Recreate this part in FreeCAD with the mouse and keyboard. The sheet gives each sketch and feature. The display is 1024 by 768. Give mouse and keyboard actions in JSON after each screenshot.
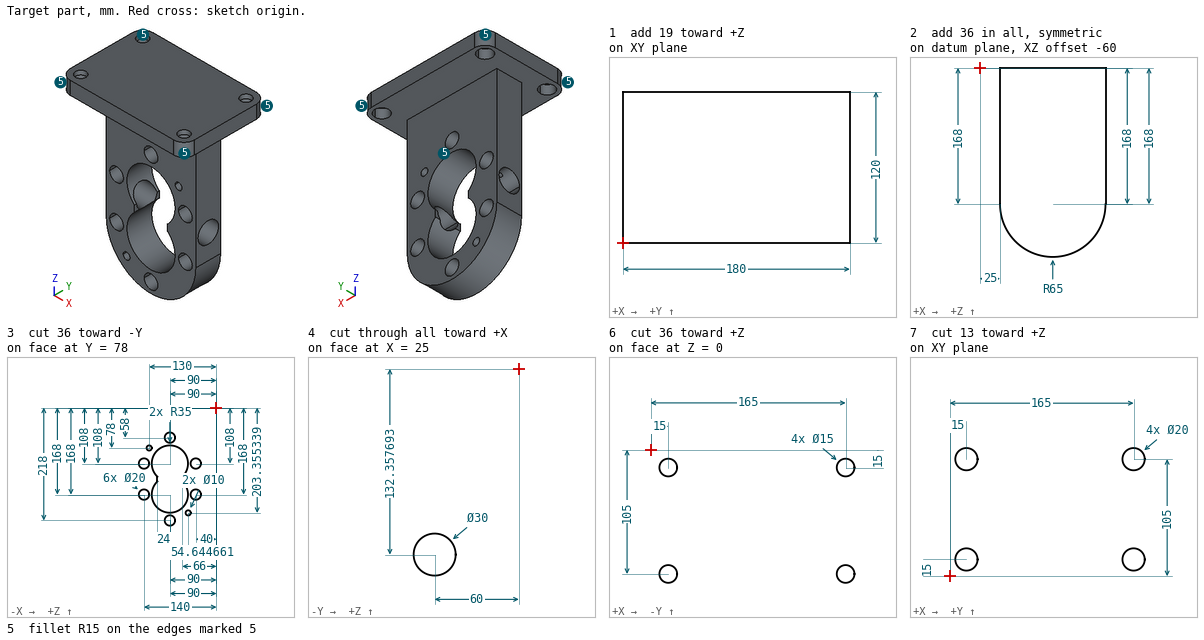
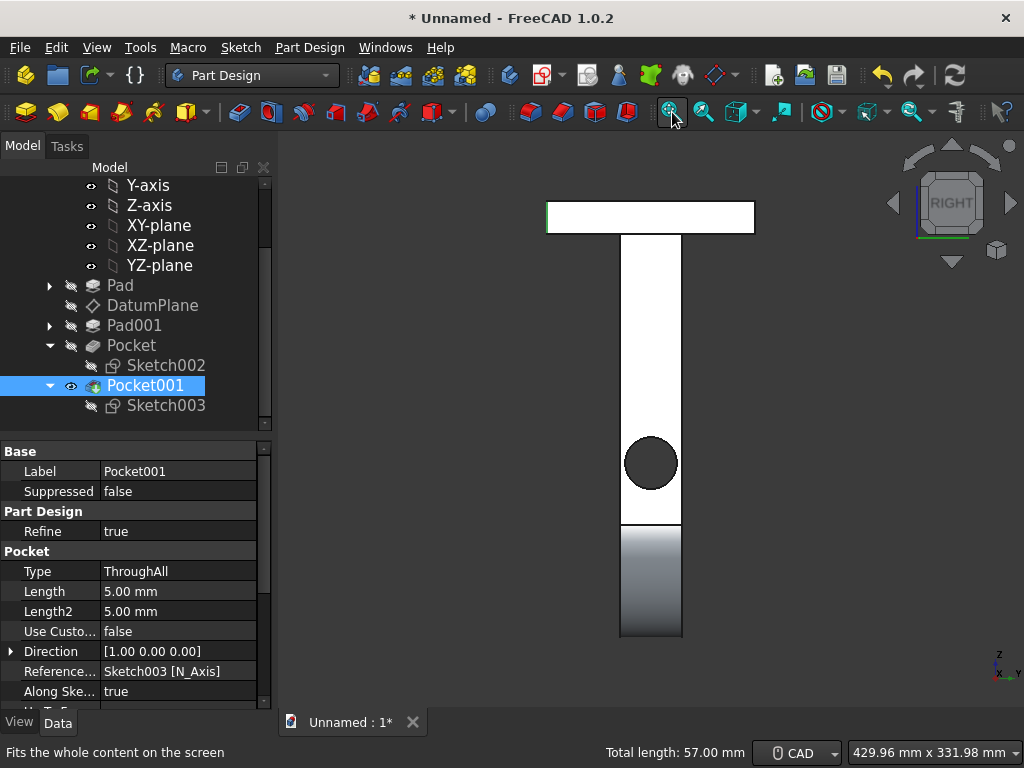
{"action": "left_click", "coordinate": [755, 216], "text": "ctrl"}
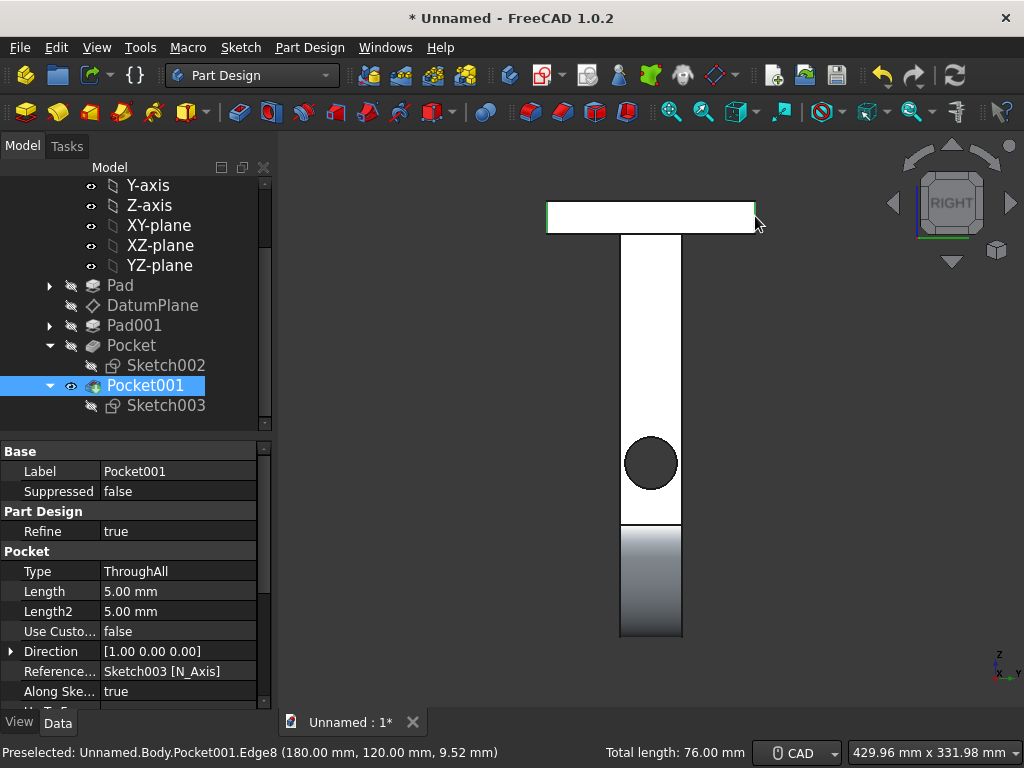
{"action": "left_click", "coordinate": [532, 112]}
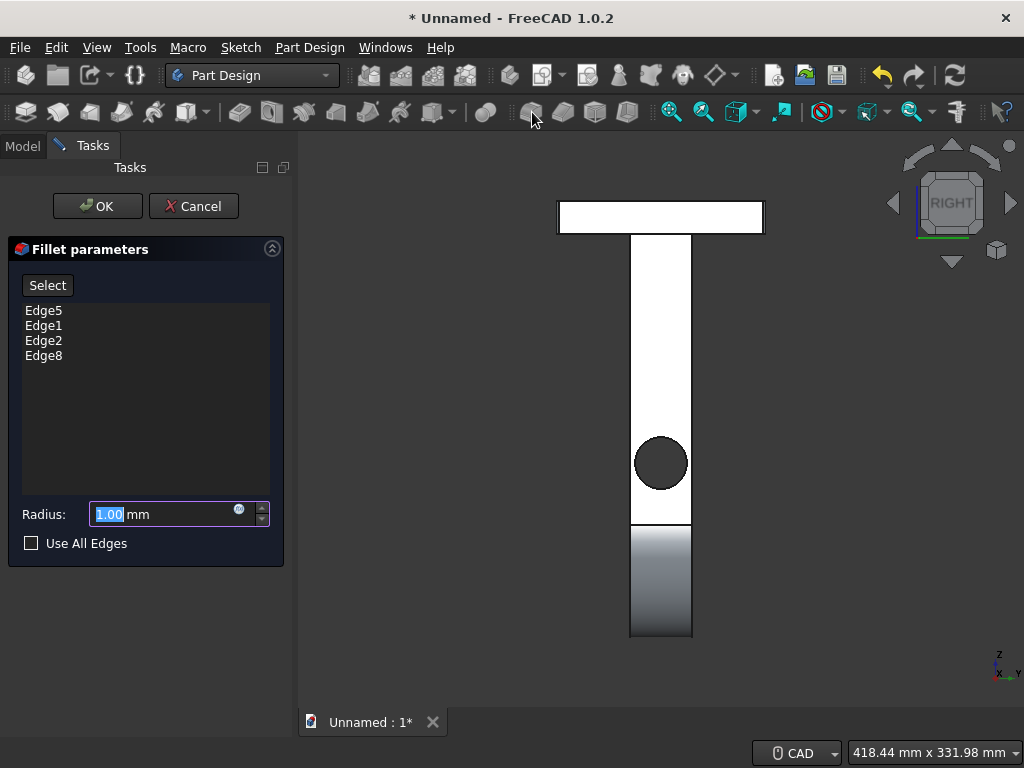
{"action": "type", "text": "15"}
{"action": "key", "text": "Tab"}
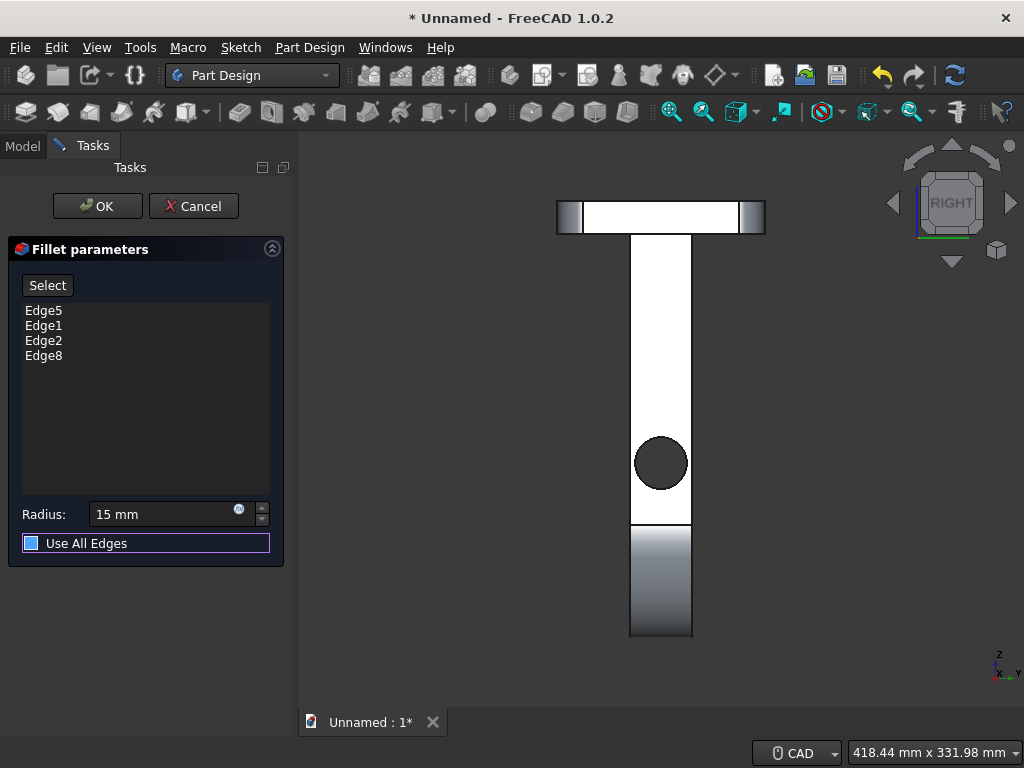
{"action": "left_click", "coordinate": [98, 206]}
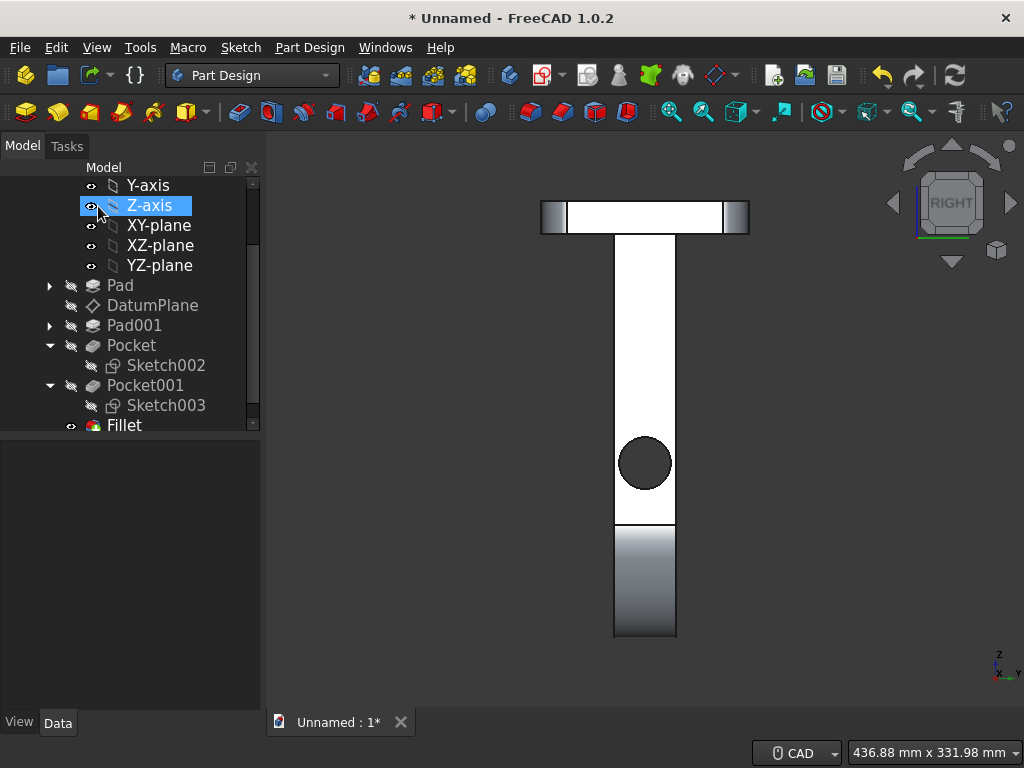
{"action": "key", "text": "5"}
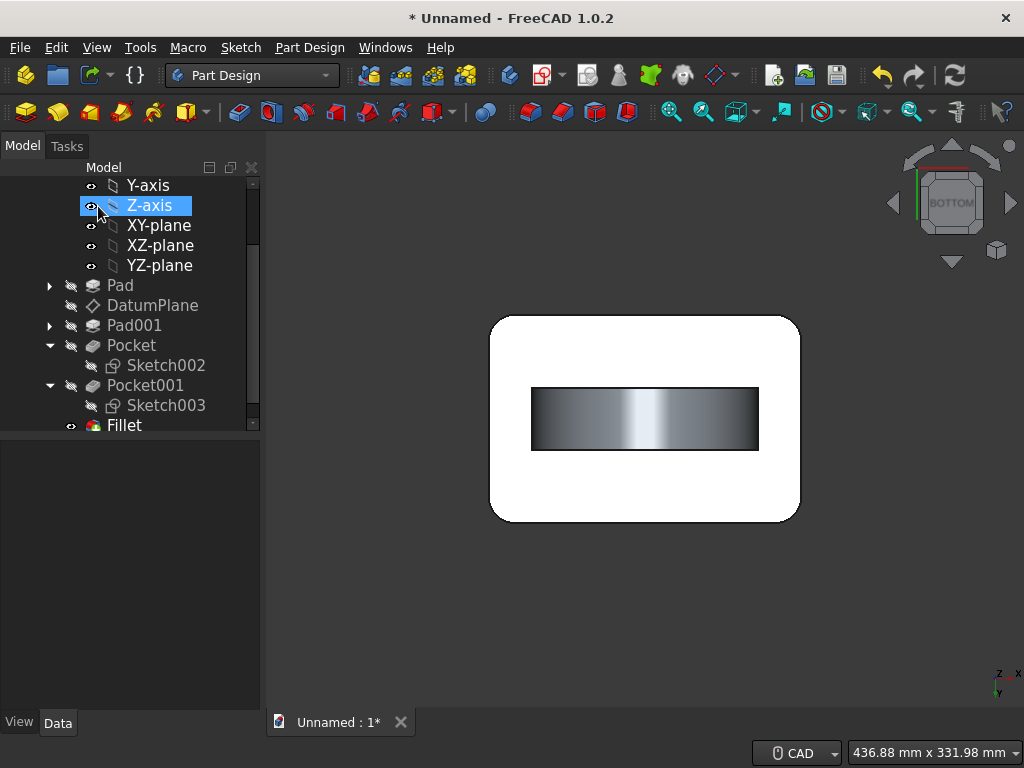
{"action": "left_click", "coordinate": [672, 112]}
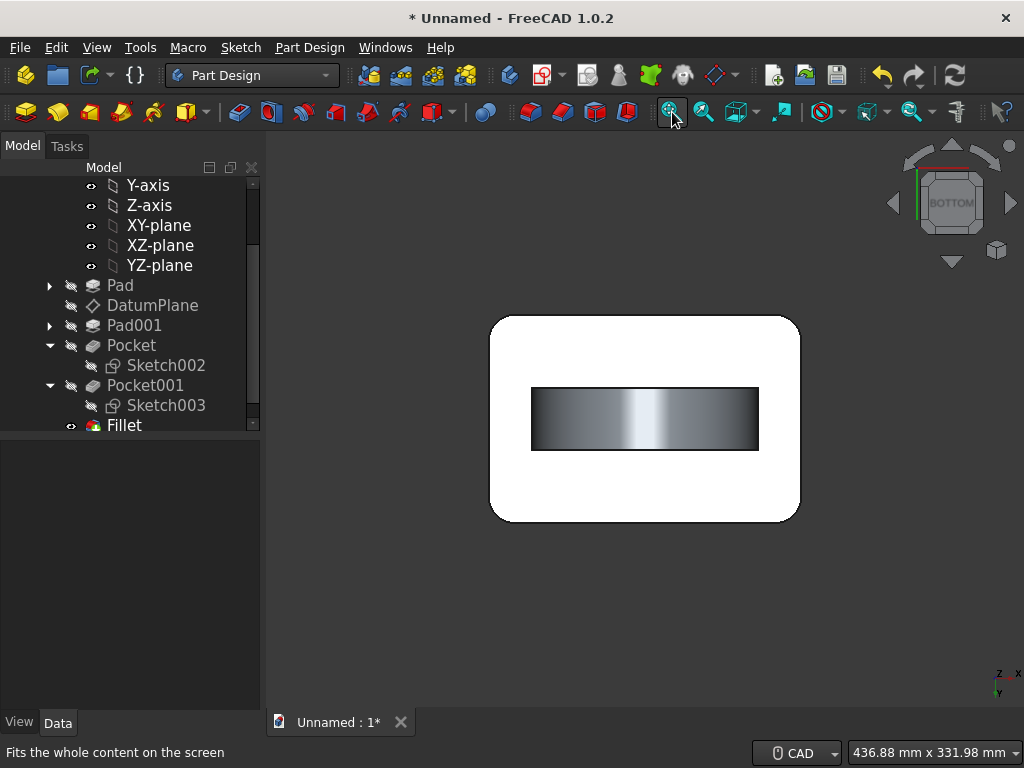
{"action": "left_click", "coordinate": [734, 477]}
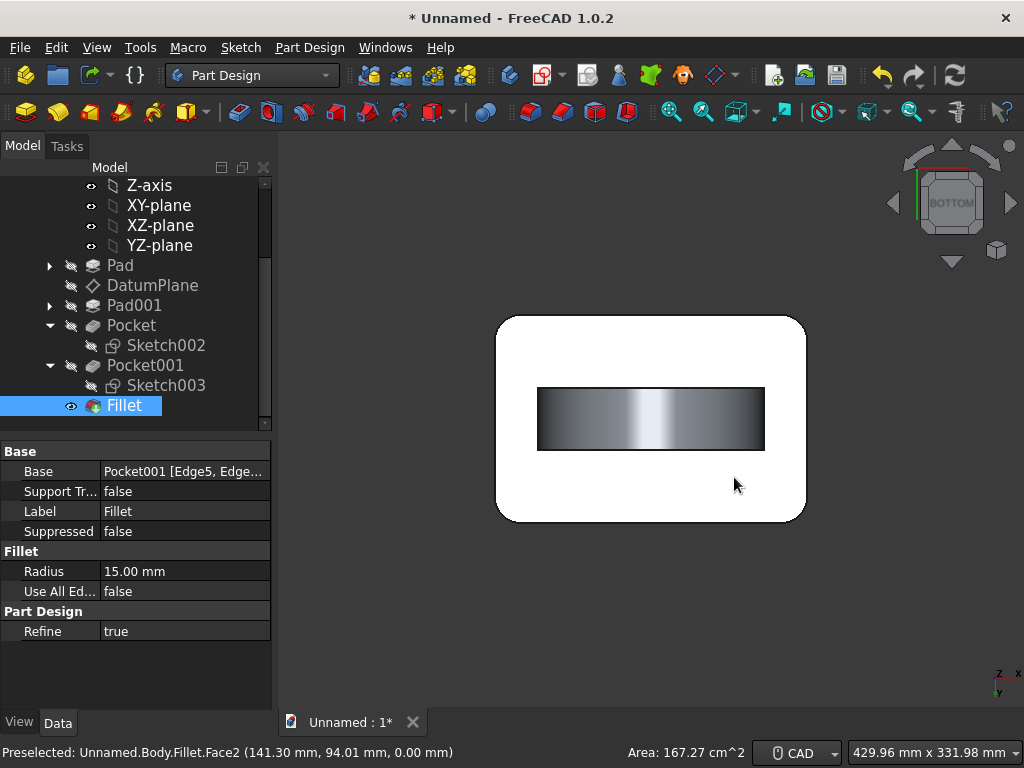
{"action": "left_click", "coordinate": [542, 76]}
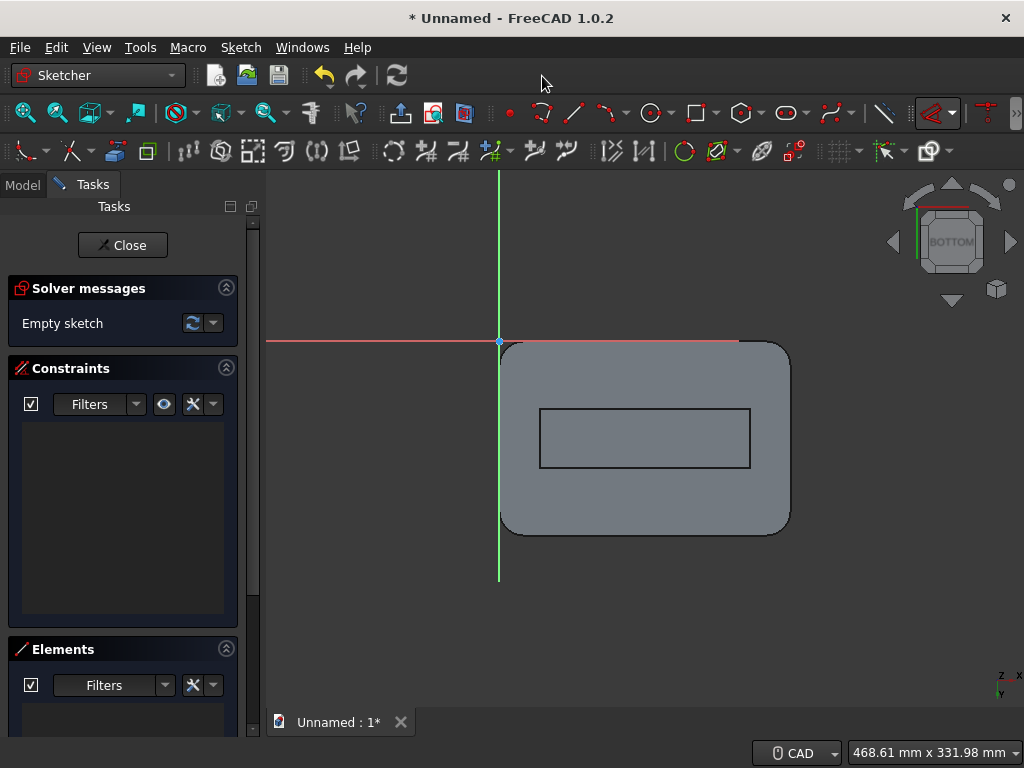
{"action": "key", "text": "q s"}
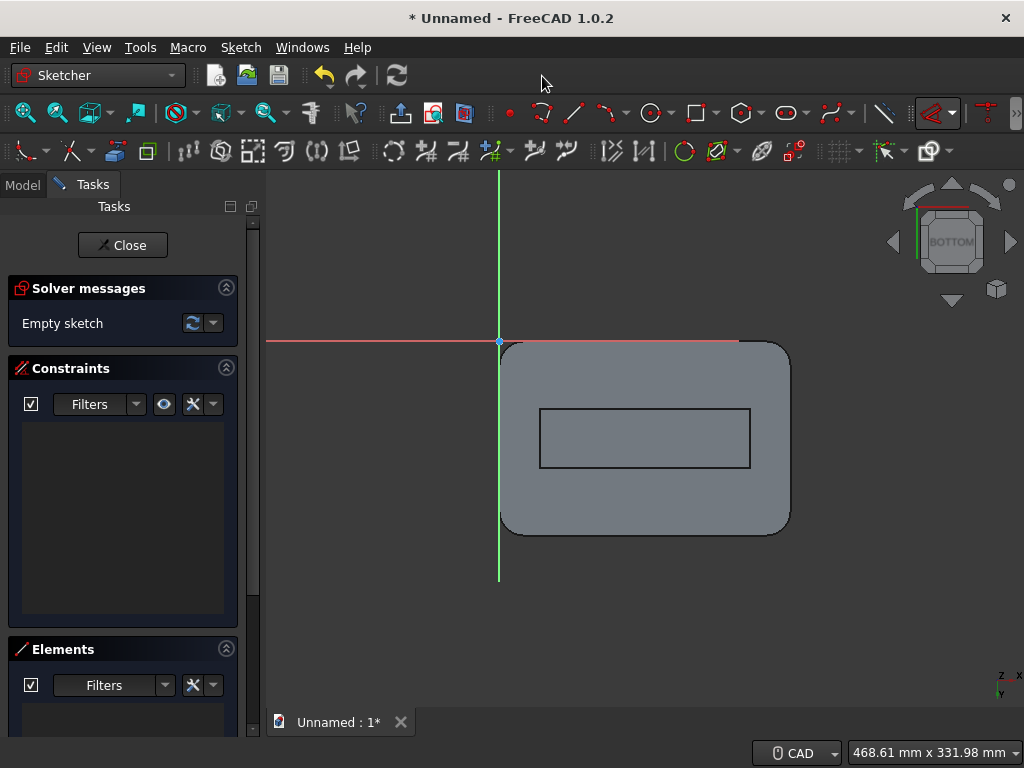
{"action": "scroll", "coordinate": [766, 420], "scroll_direction": "up", "scroll_amount": 2}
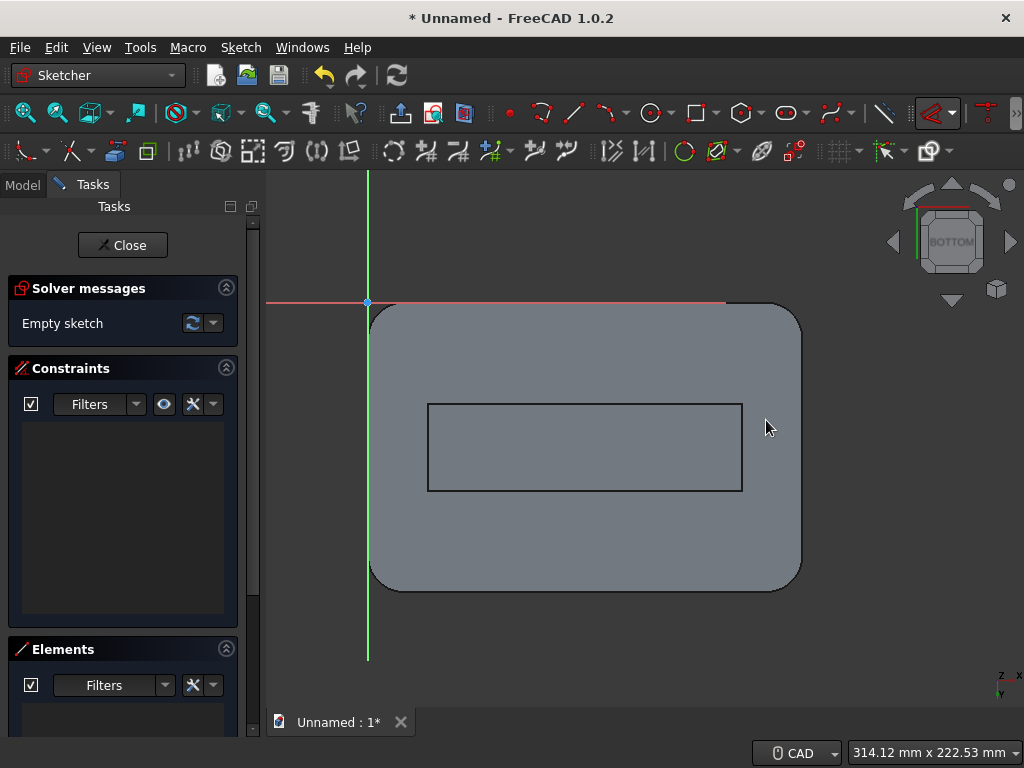
{"action": "key", "text": "g c"}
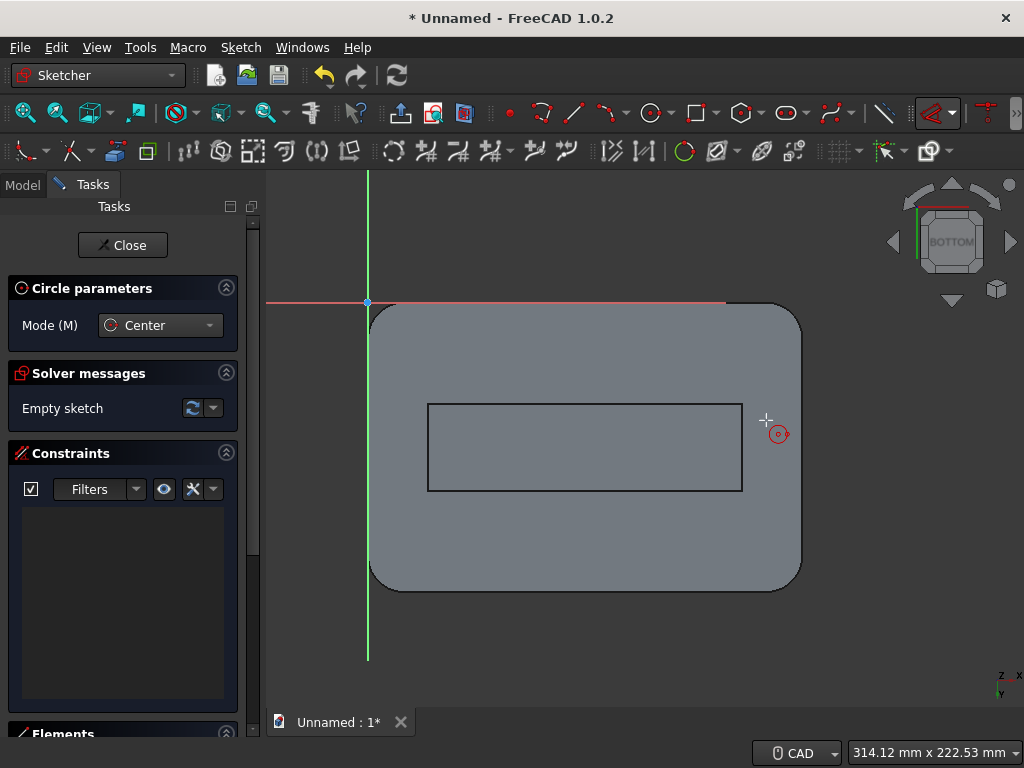
{"action": "scroll", "coordinate": [766, 339], "scroll_direction": "up", "scroll_amount": 2}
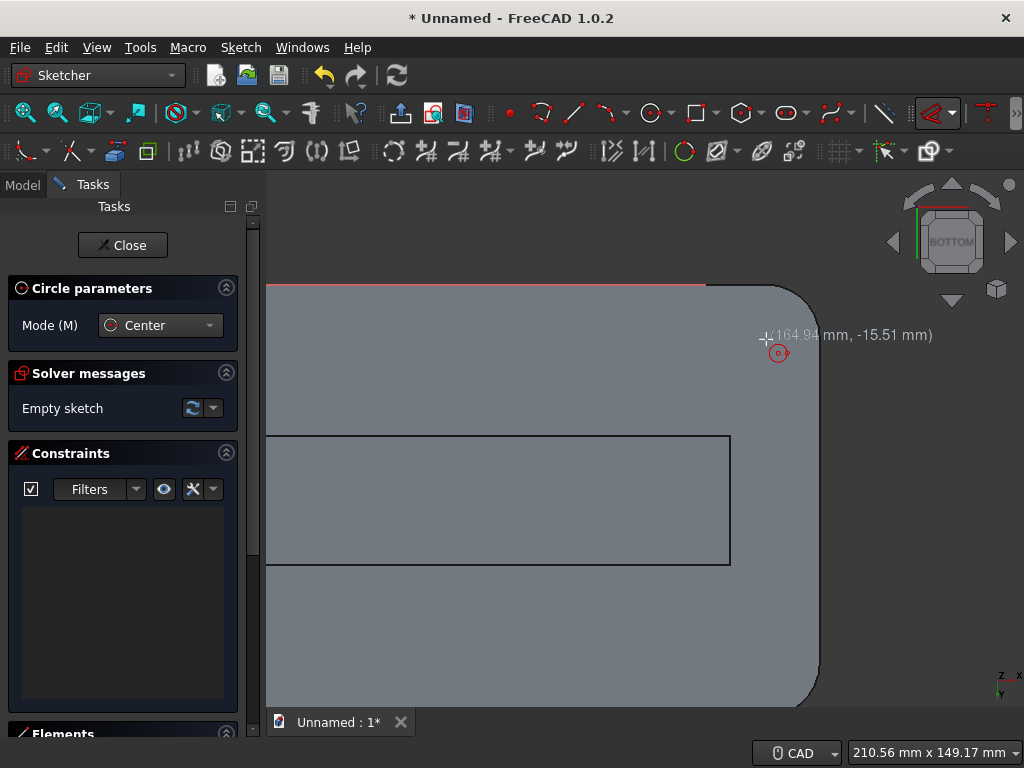
{"action": "left_click", "coordinate": [766, 339]}
{"action": "left_click", "coordinate": [785, 319]}